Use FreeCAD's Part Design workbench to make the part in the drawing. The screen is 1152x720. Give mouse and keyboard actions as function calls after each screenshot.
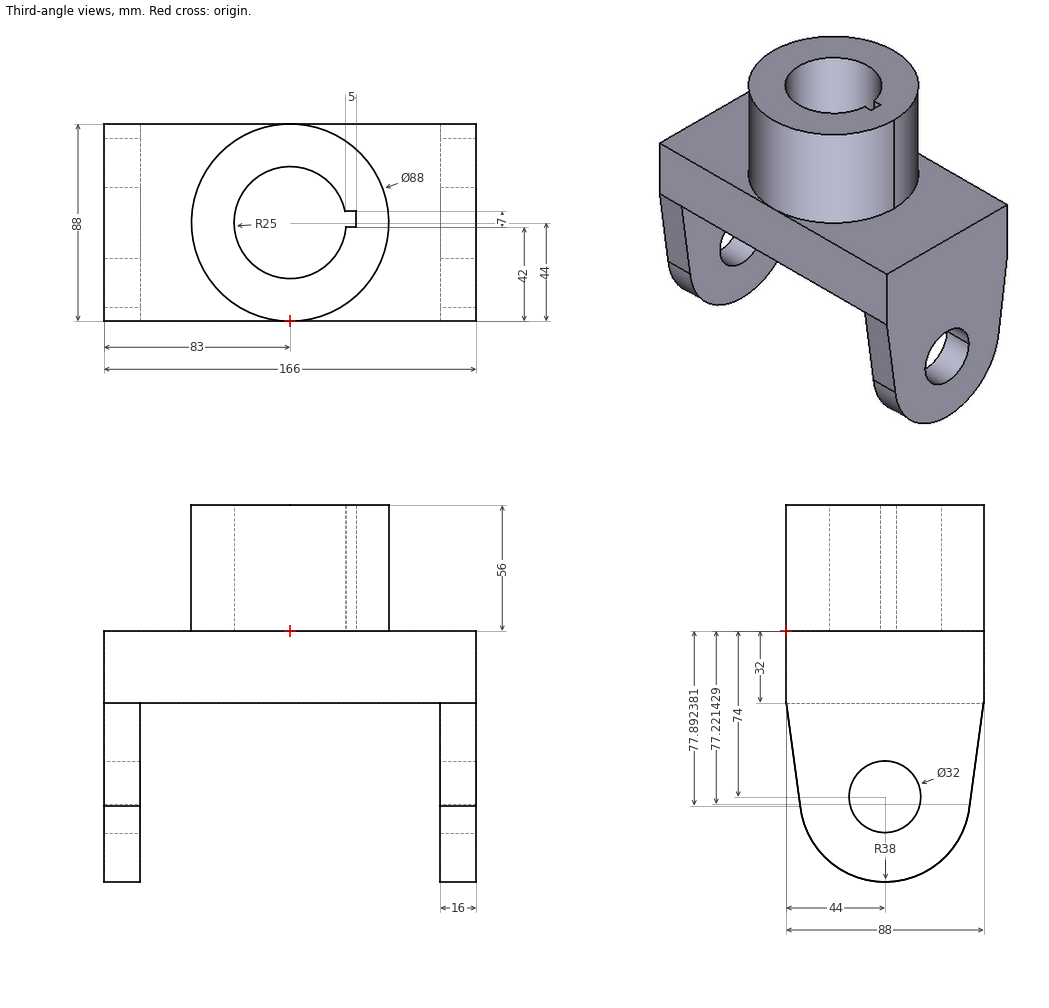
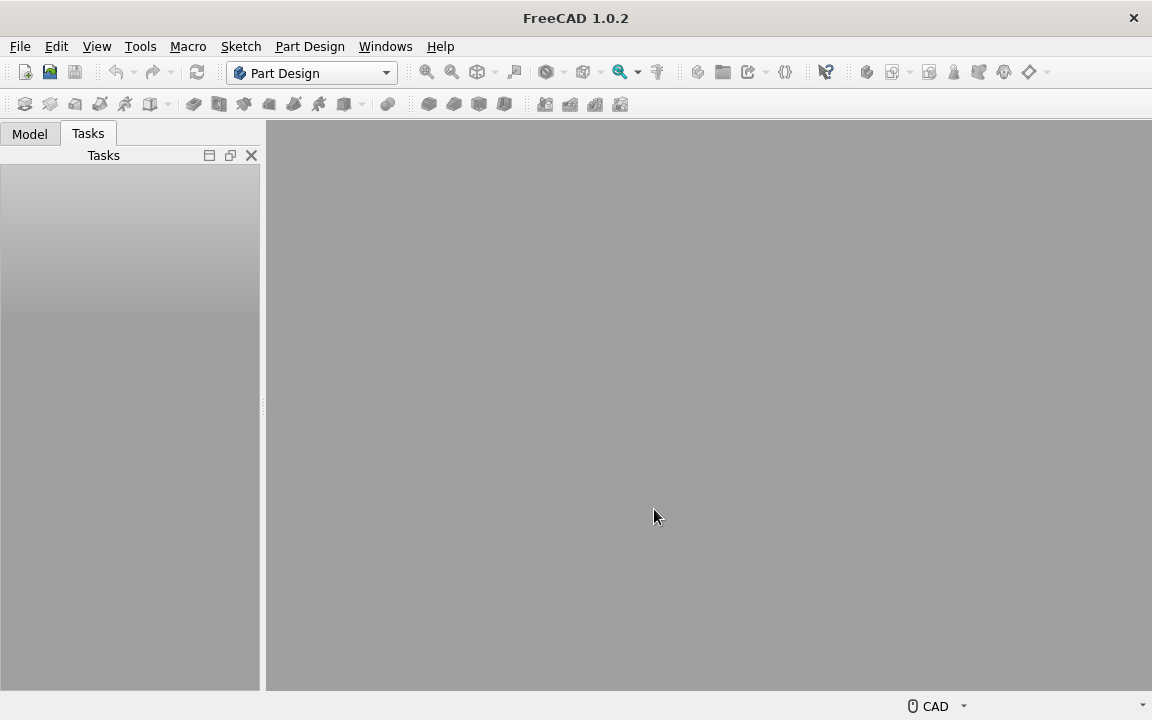
click(25, 72)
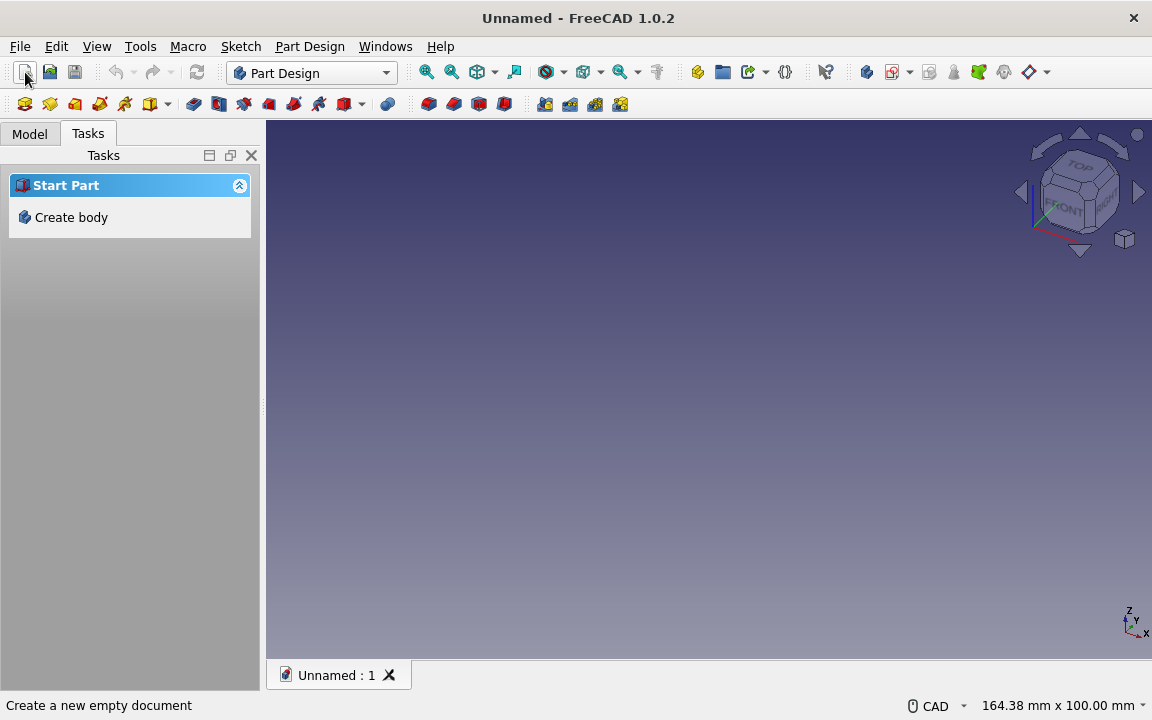
click(892, 72)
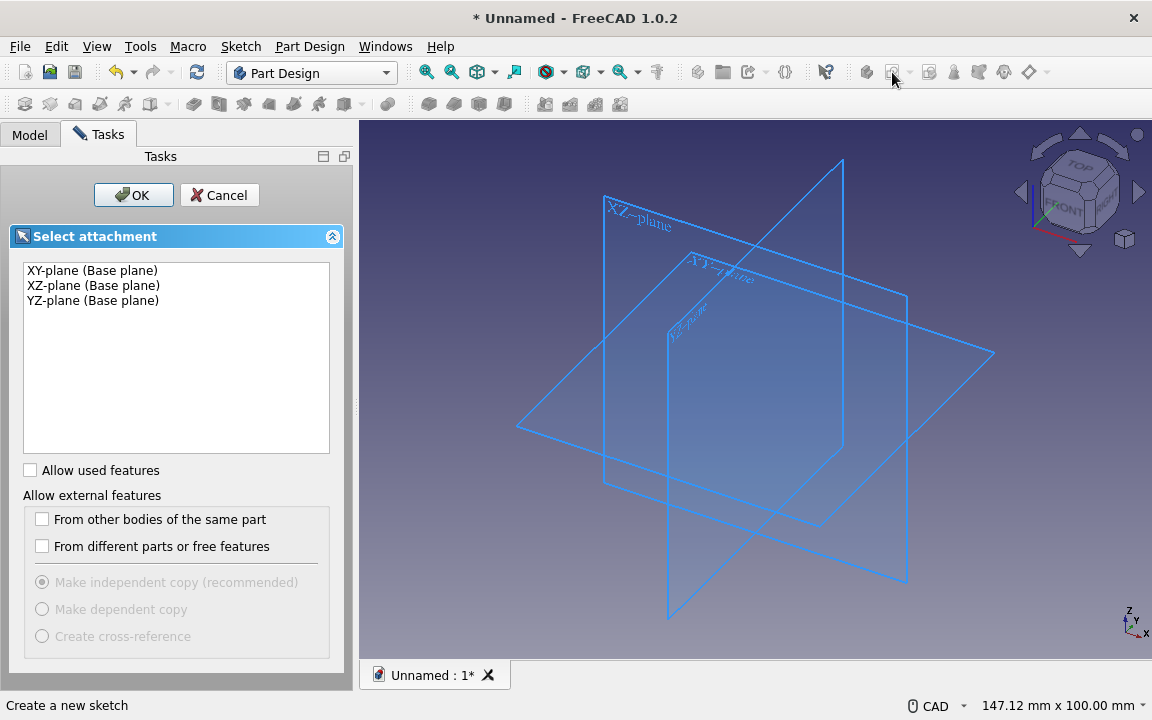
click(84, 270)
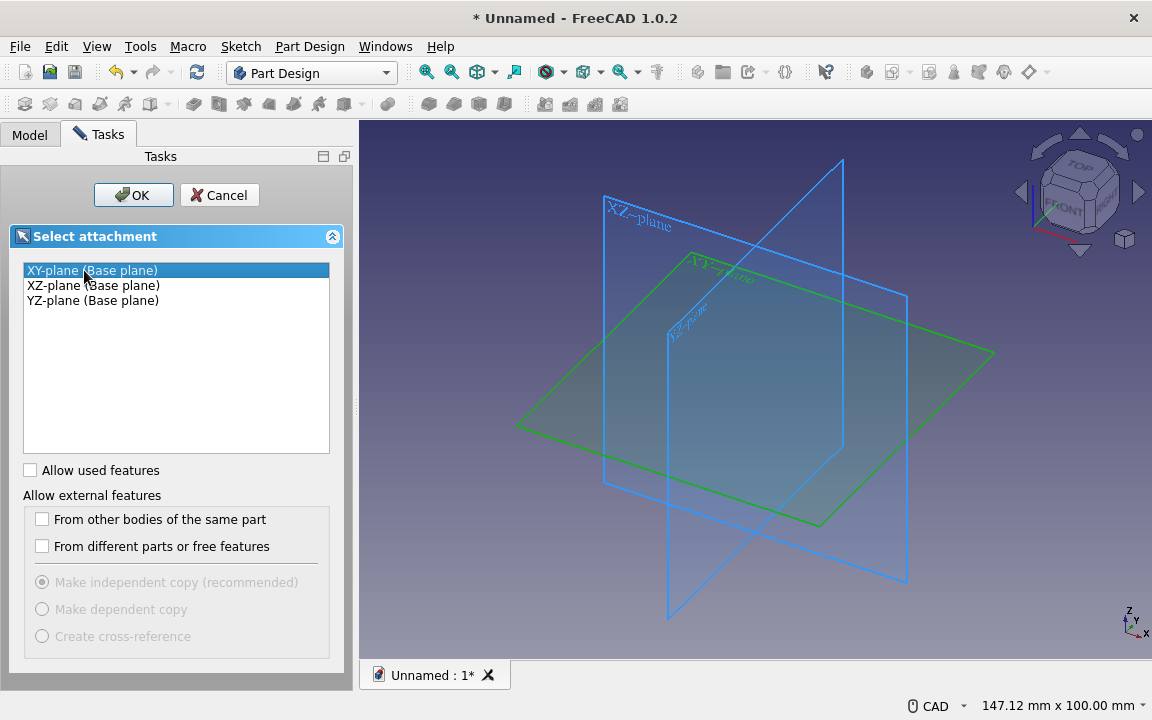
click(134, 195)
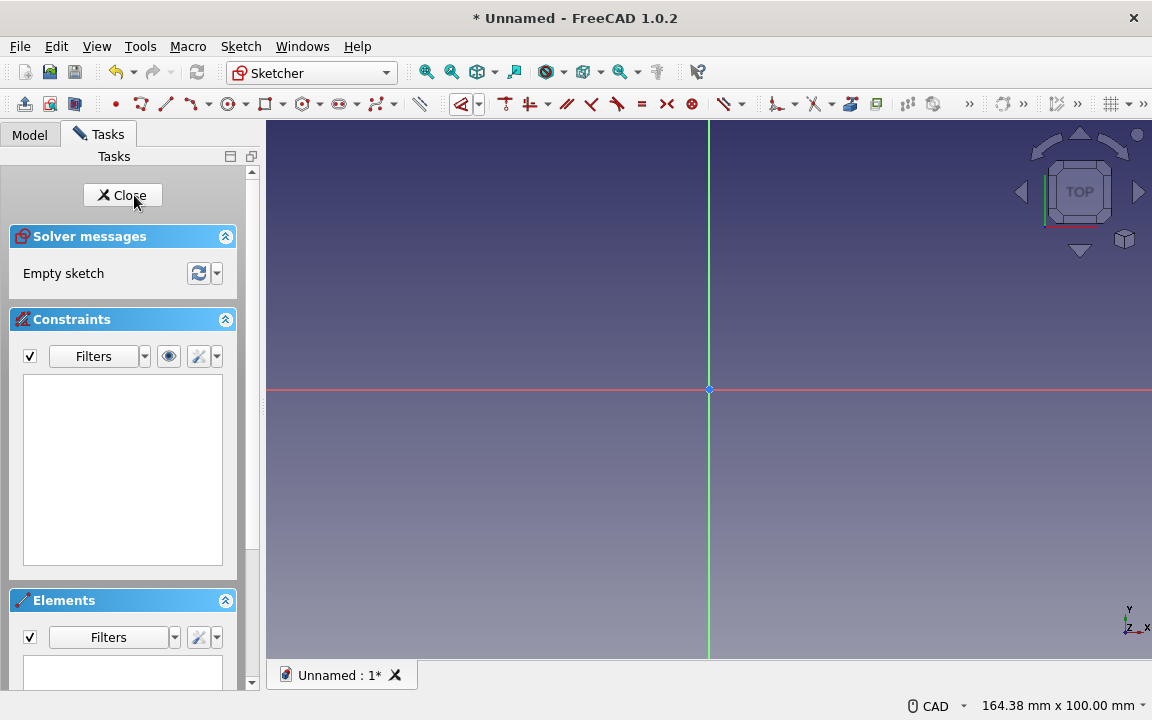
scroll(557, 631, down, 3)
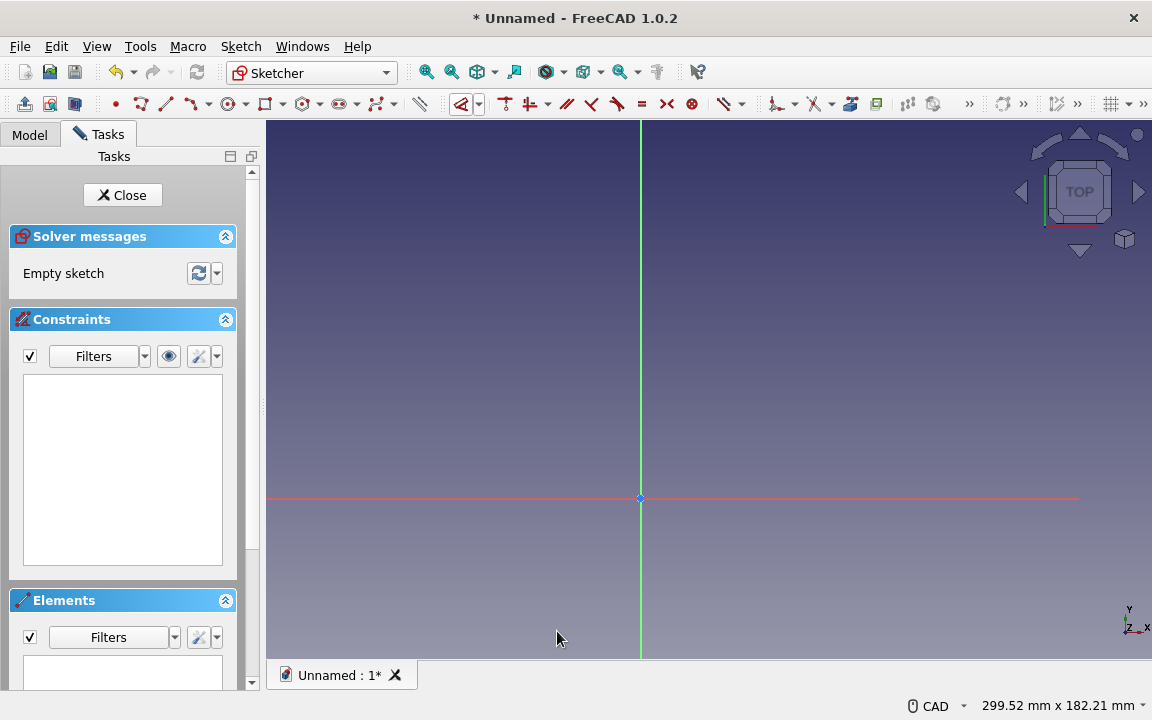
click(264, 104)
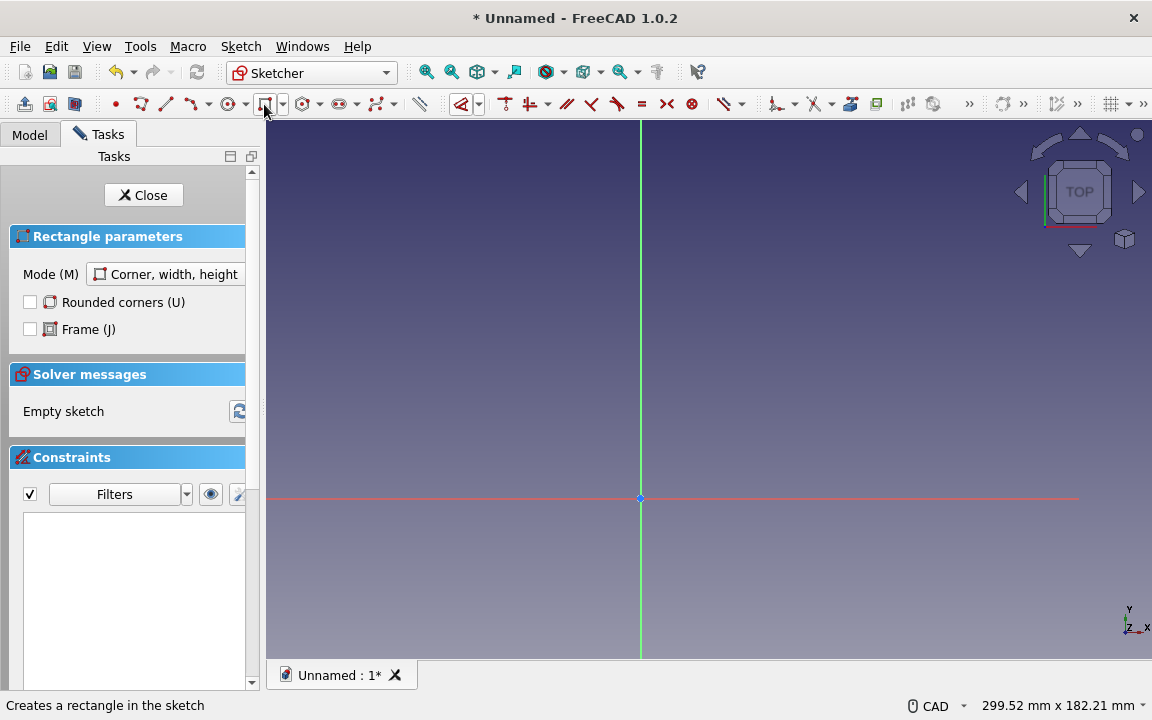
click(395, 239)
click(886, 499)
key(Escape)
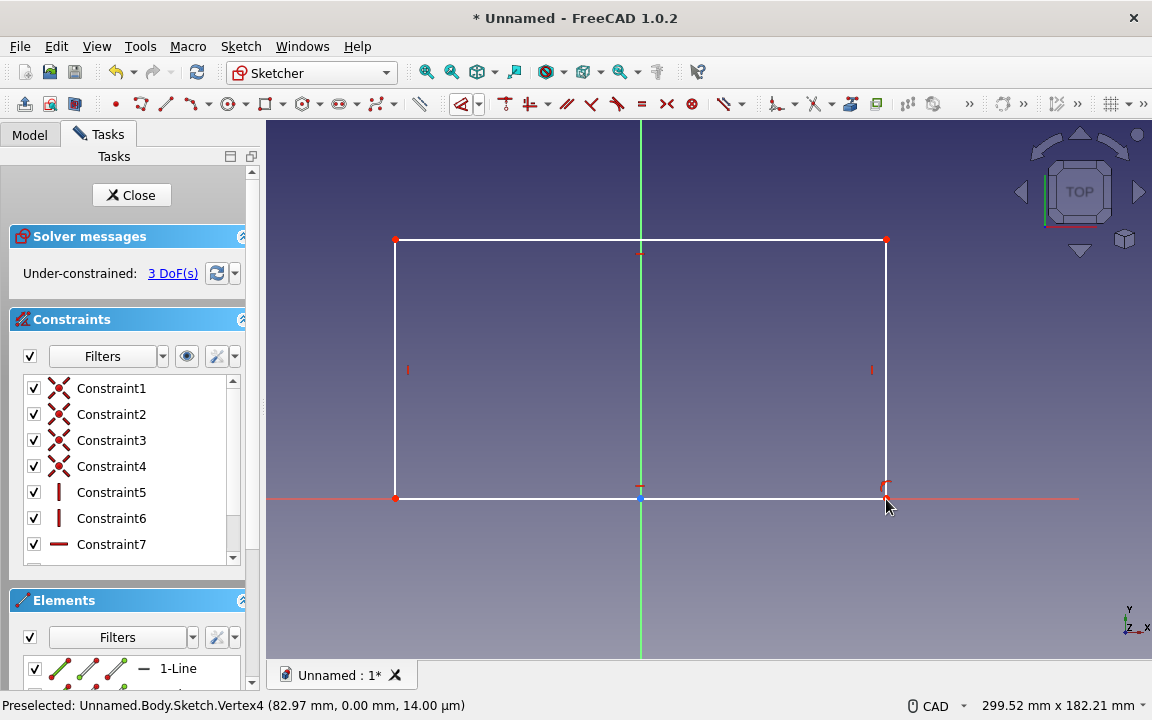
click(460, 104)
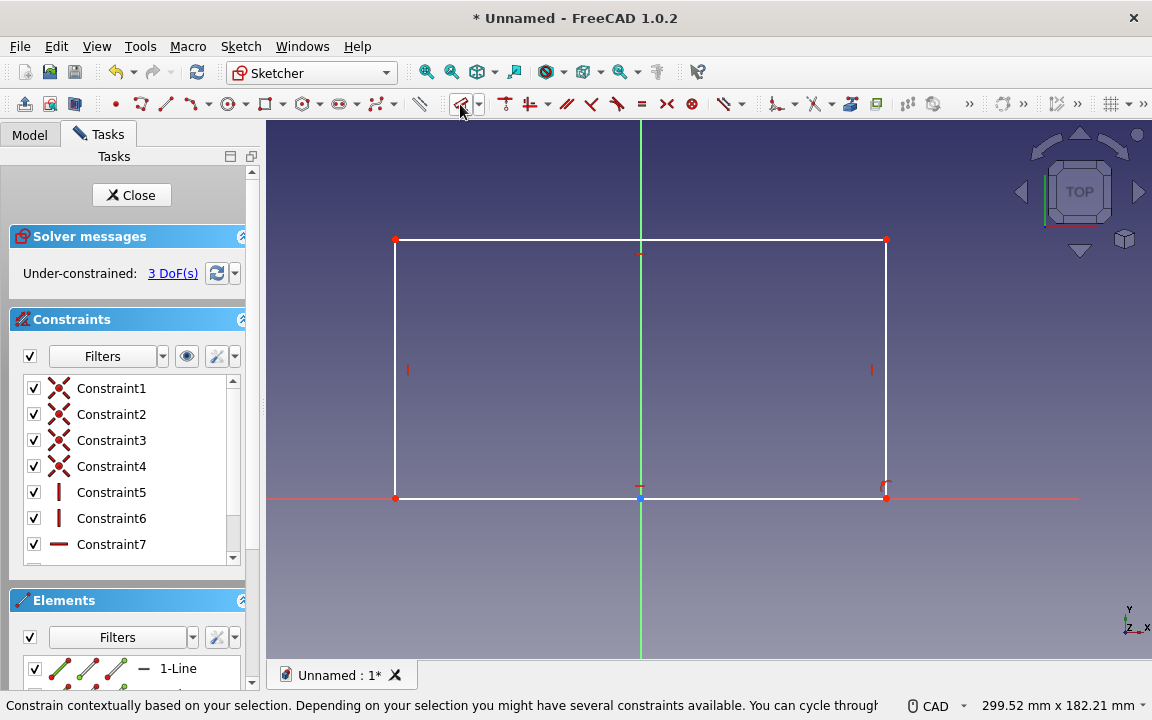
click(395, 318)
click(361, 369)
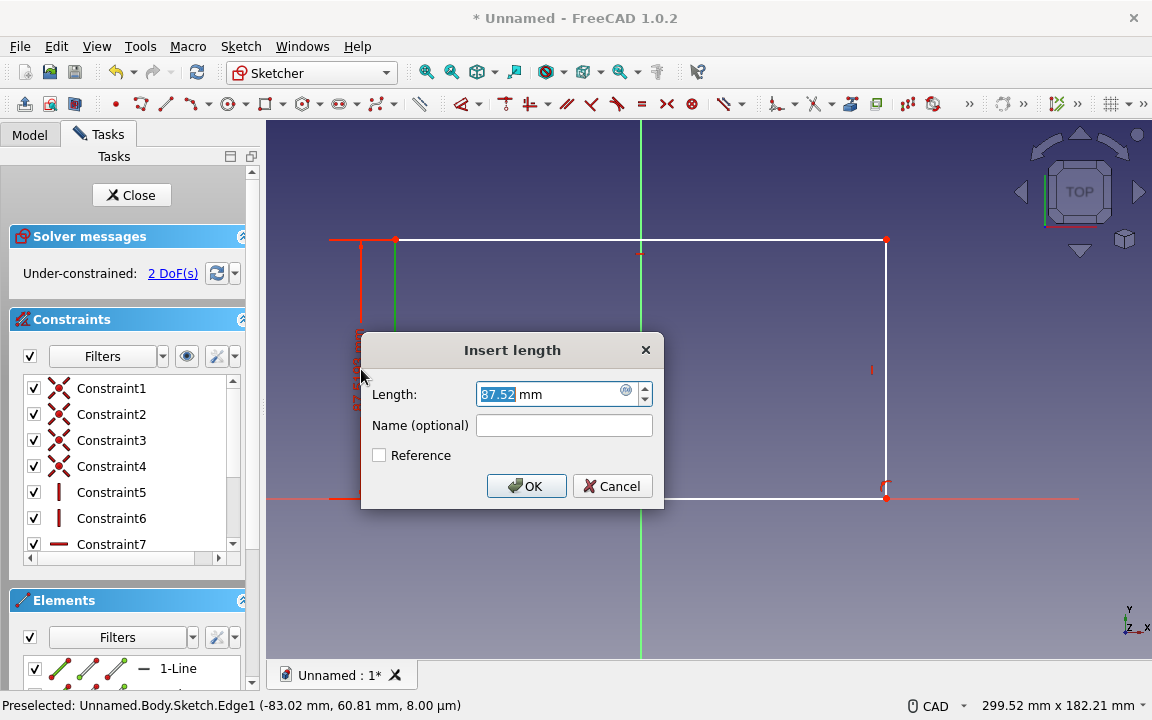
text(88)
key(Return)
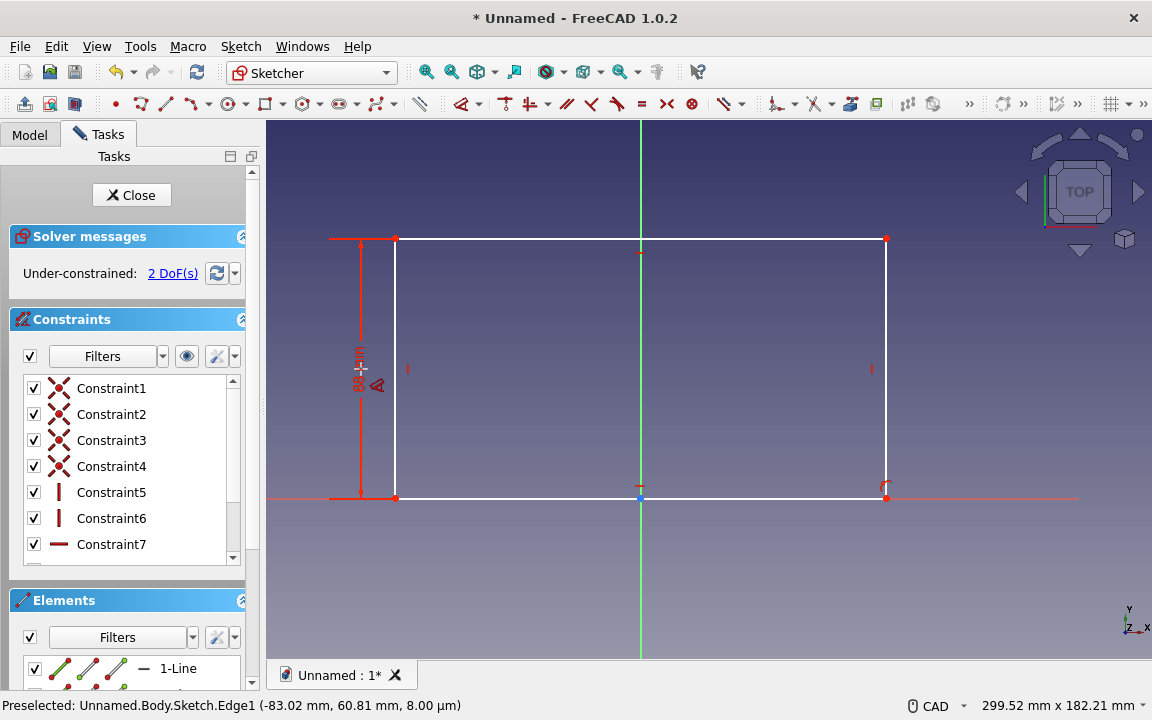
click(542, 499)
click(528, 533)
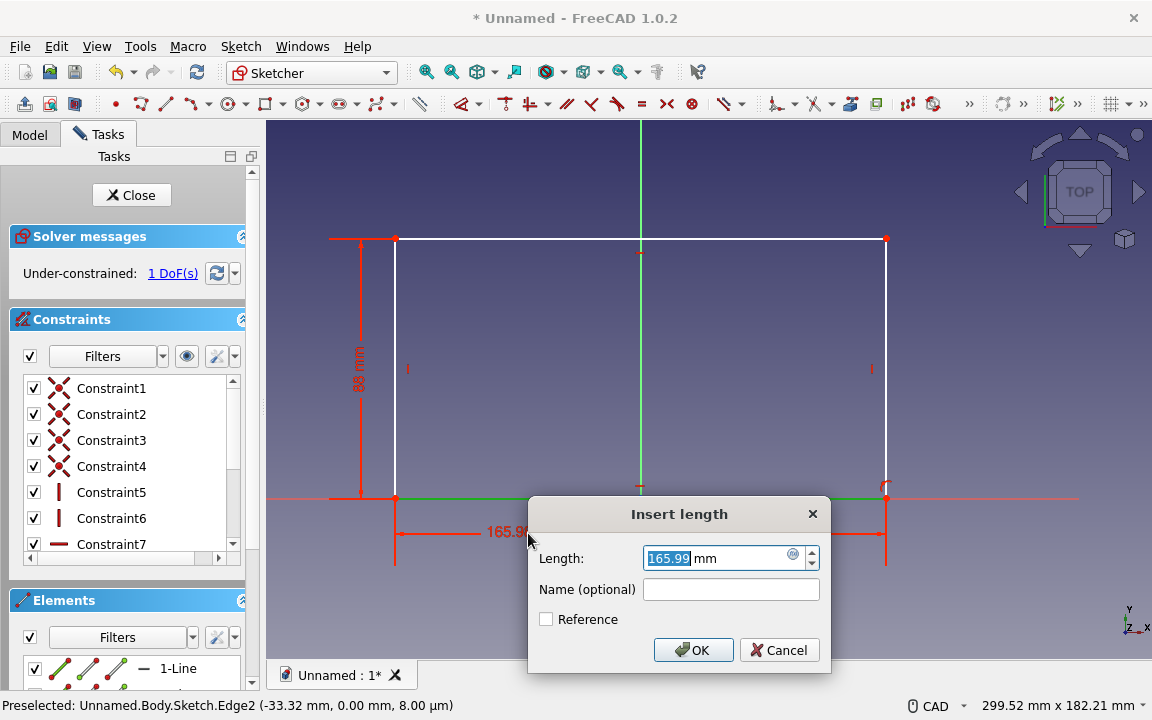
text(166)
key(Return)